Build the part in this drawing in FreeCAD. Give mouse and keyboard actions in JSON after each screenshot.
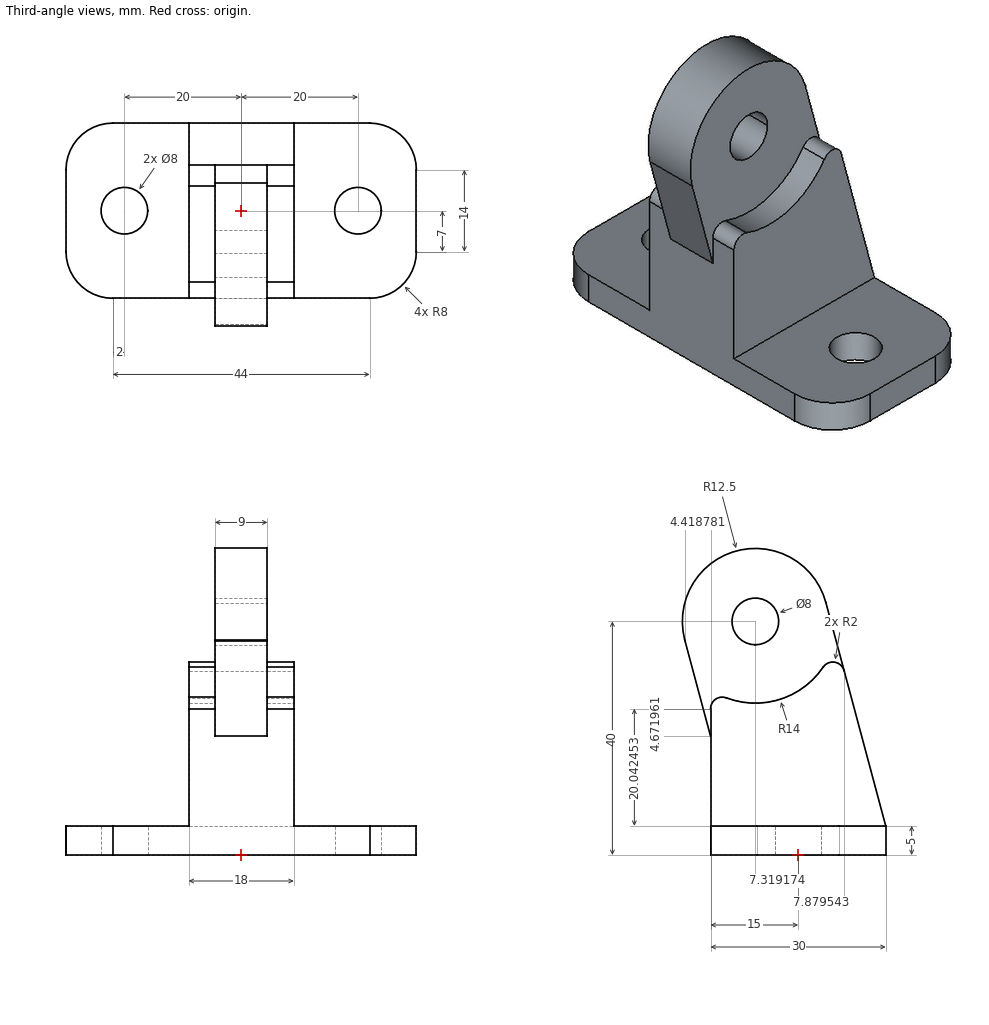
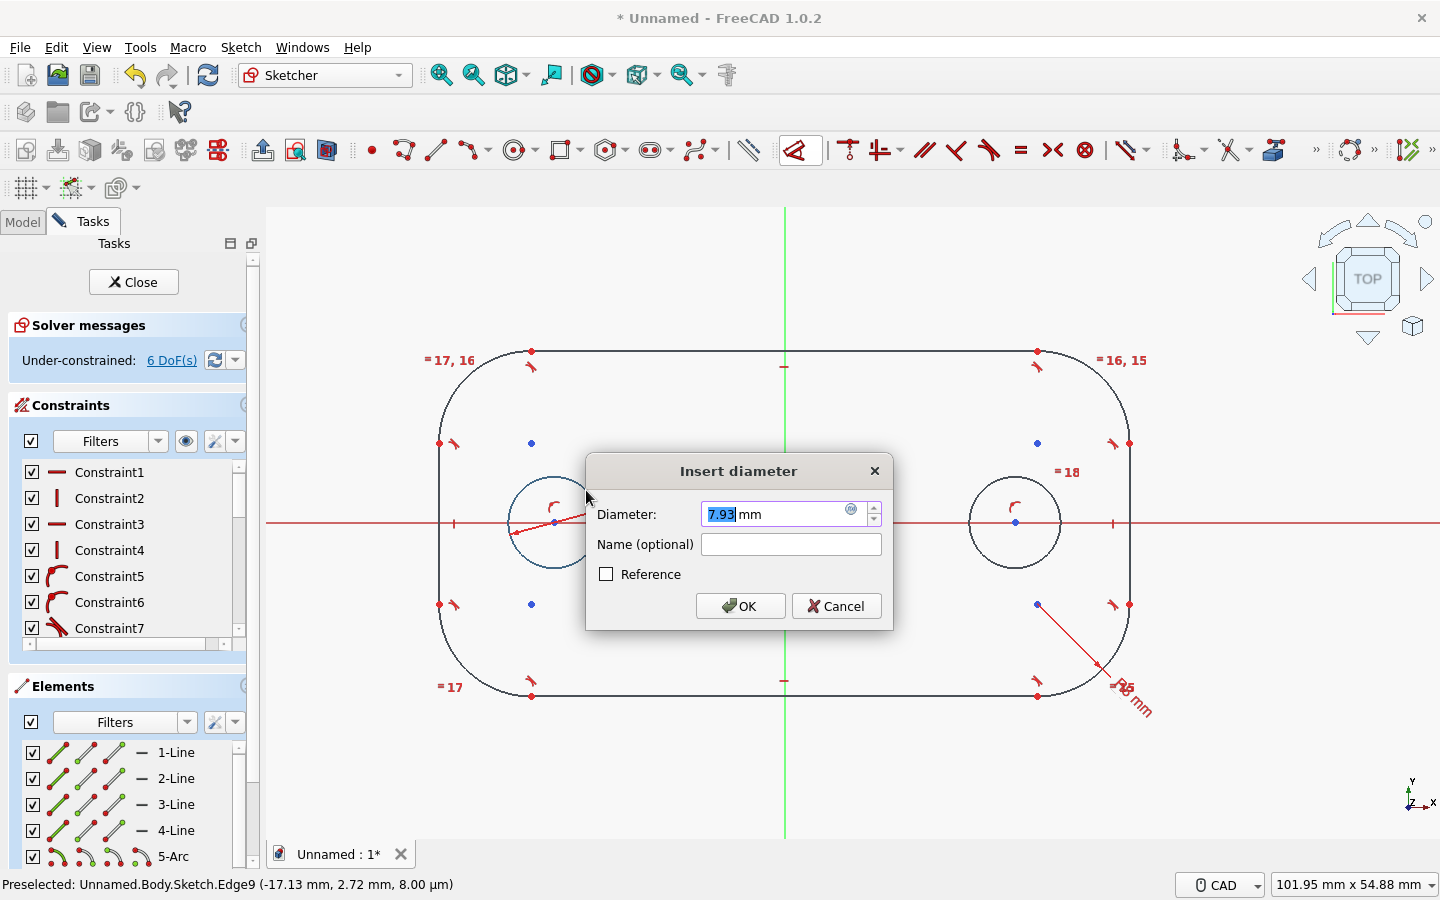
{"action": "type", "text": "8"}
{"action": "key", "text": "Return"}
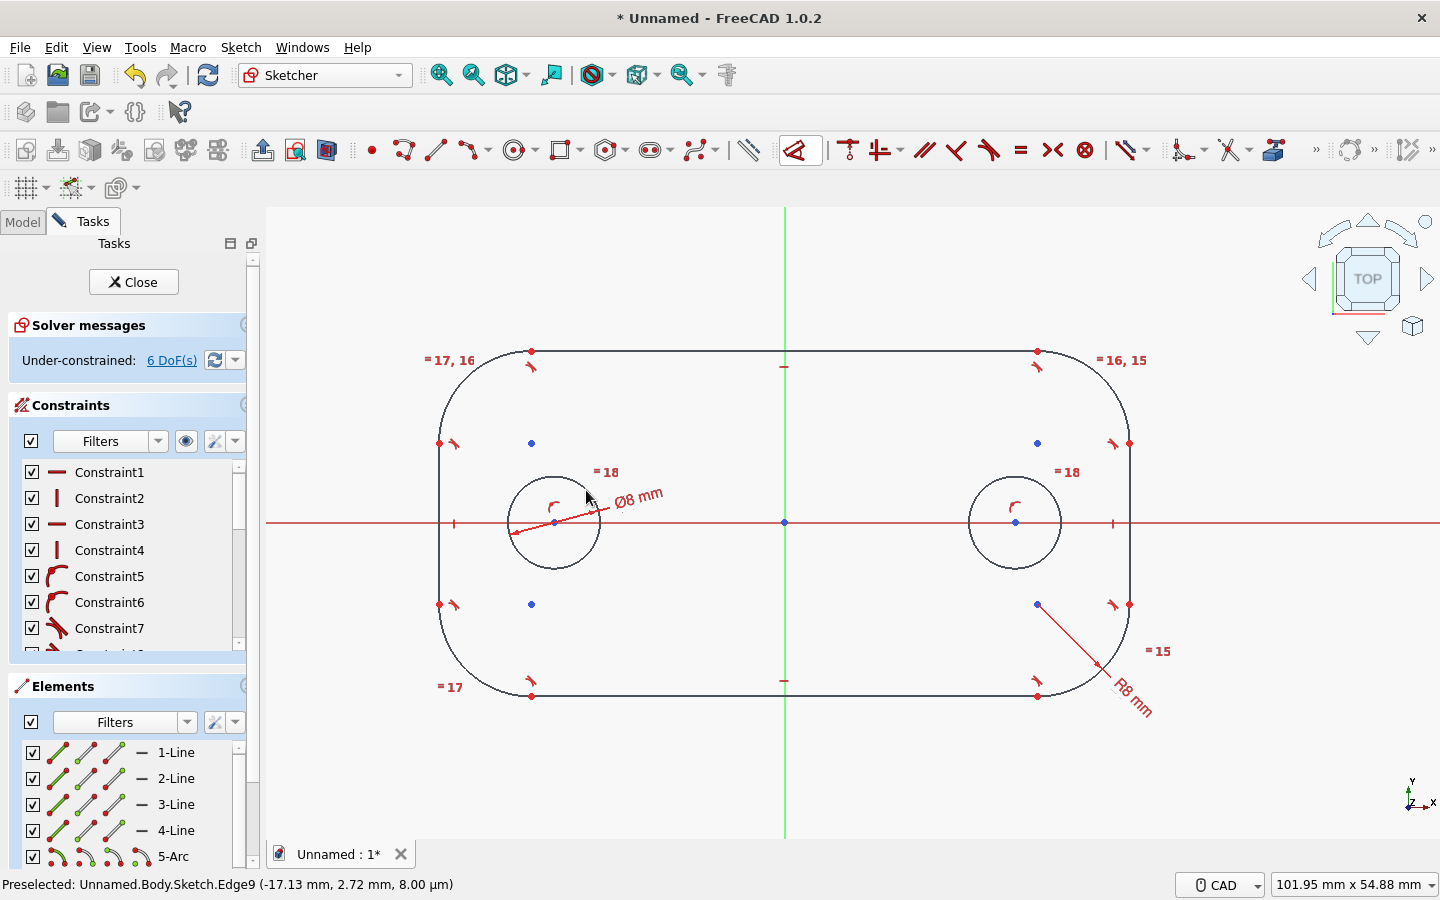
{"action": "left_click", "coordinate": [683, 696]}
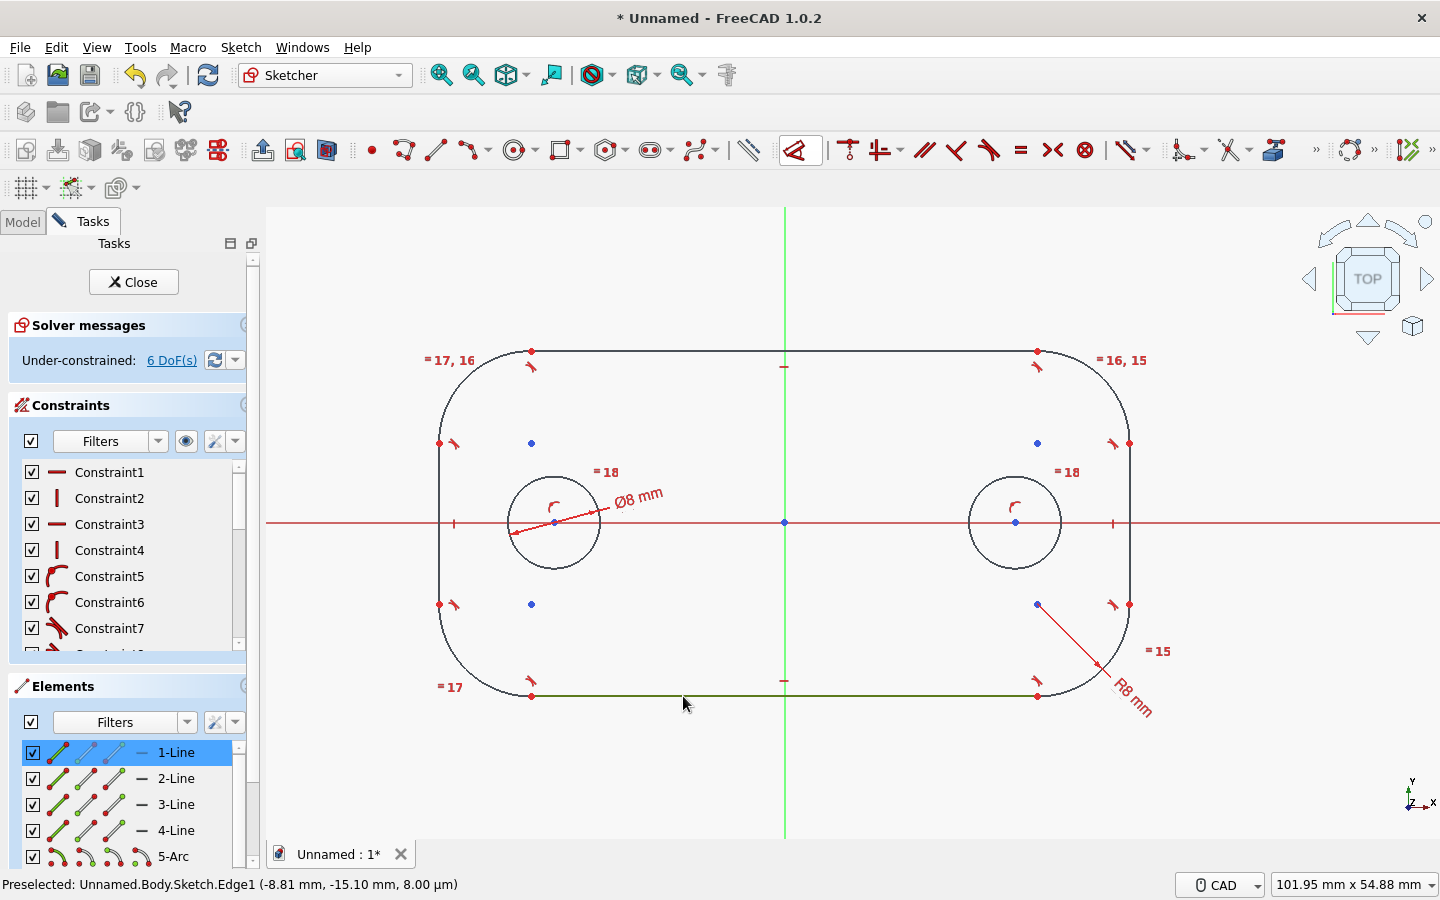
{"action": "key", "text": "l"}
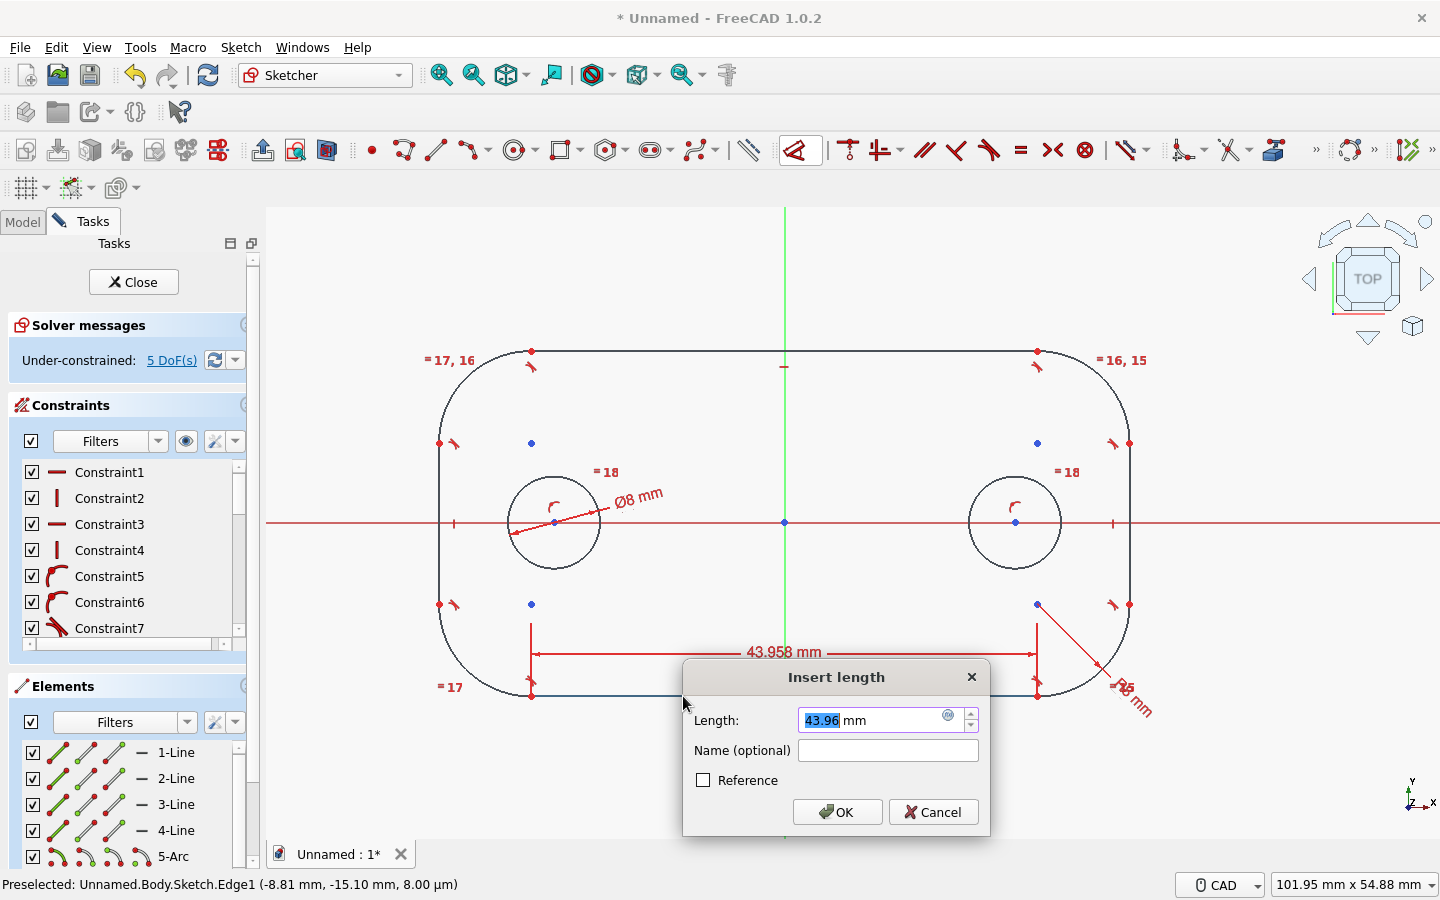
{"action": "type", "text": "44"}
{"action": "key", "text": "Return"}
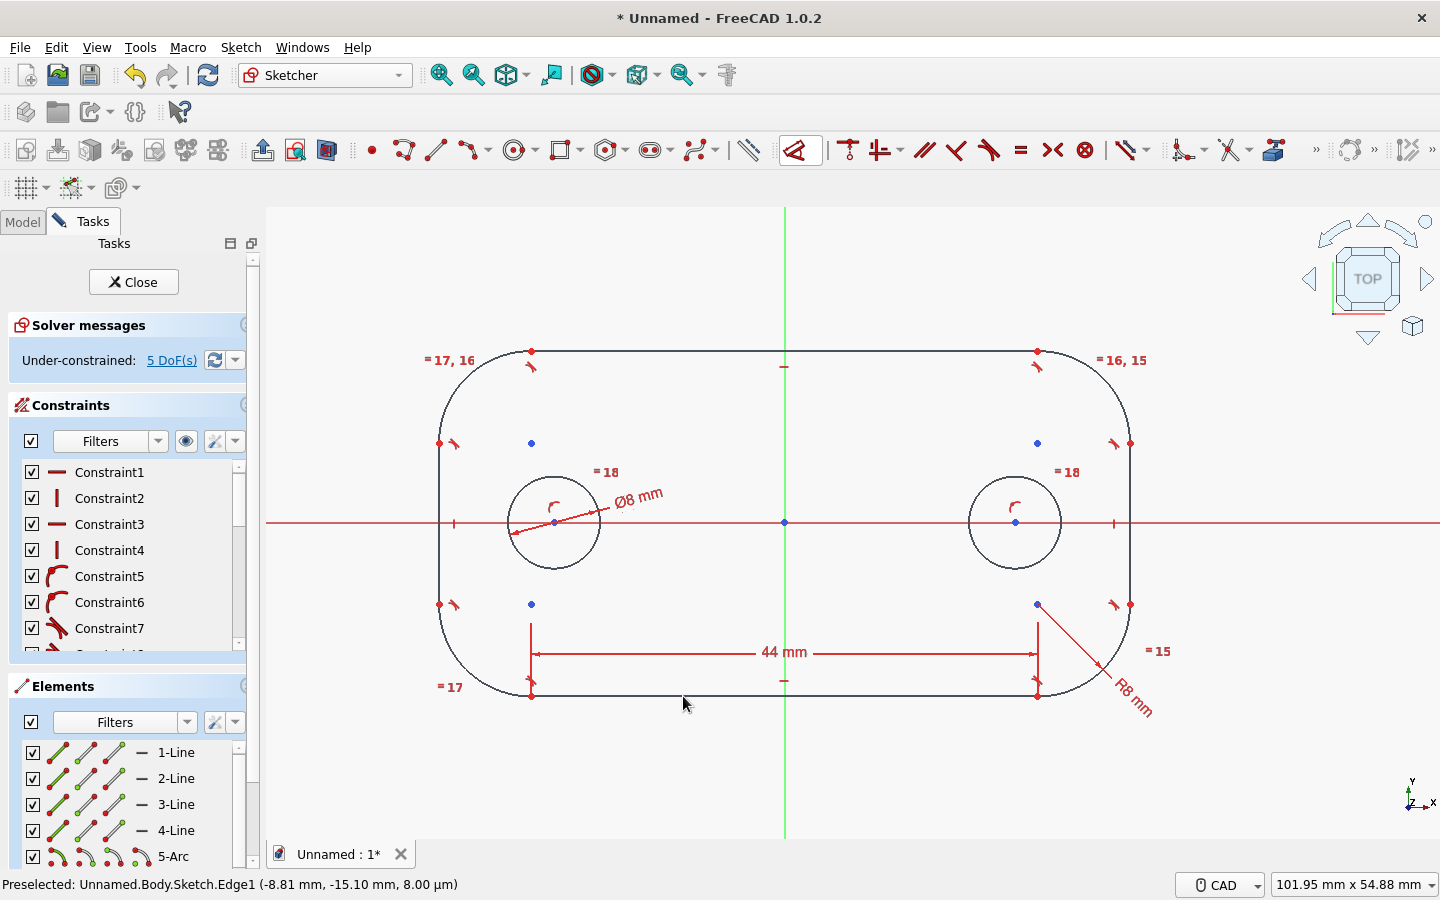
{"action": "left_click", "coordinate": [1130, 556]}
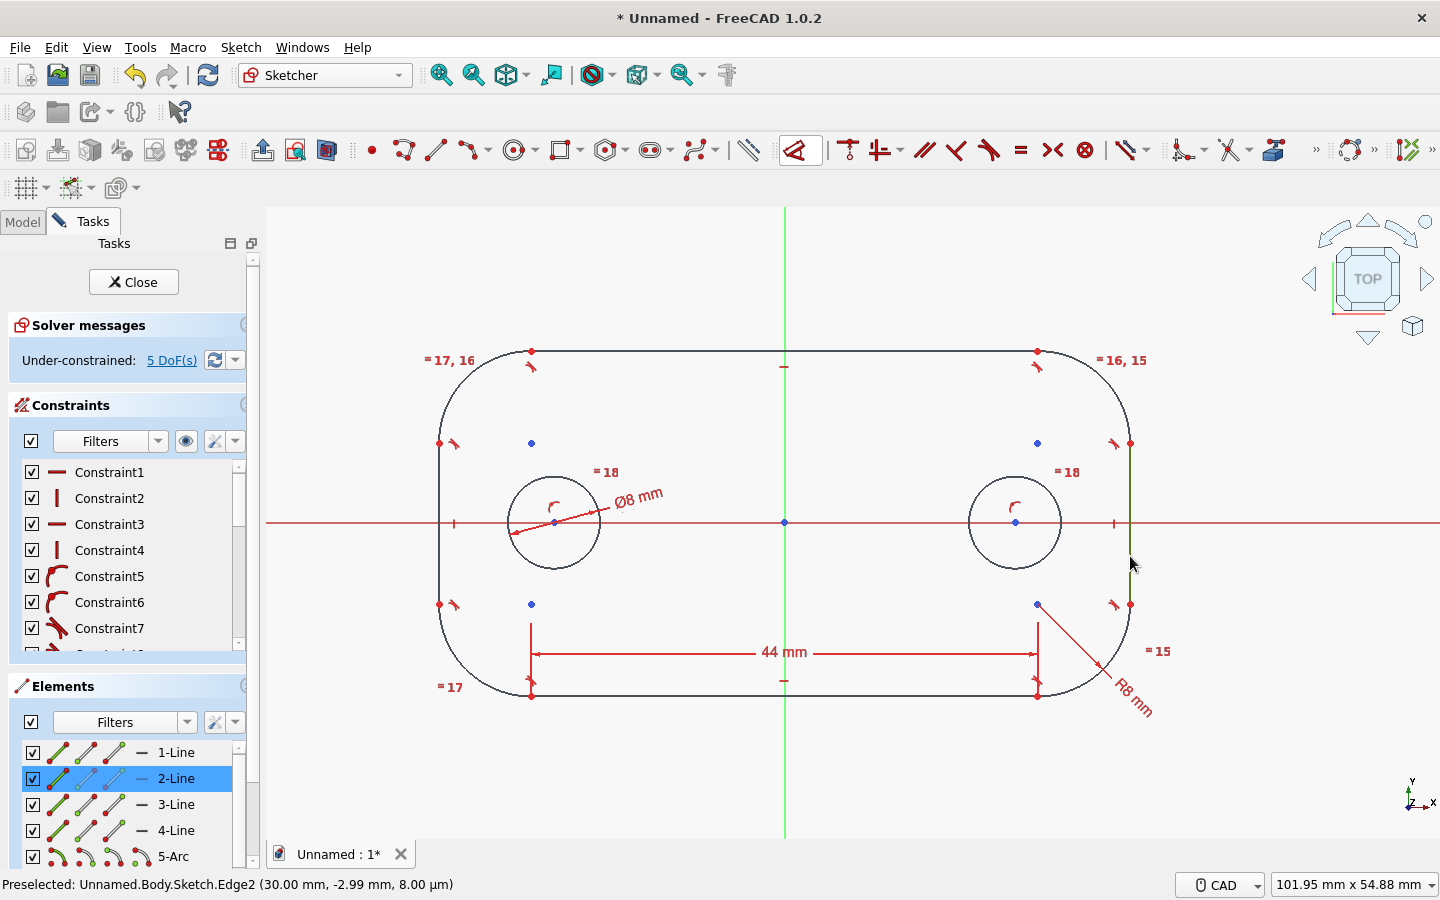
{"action": "key", "text": "i"}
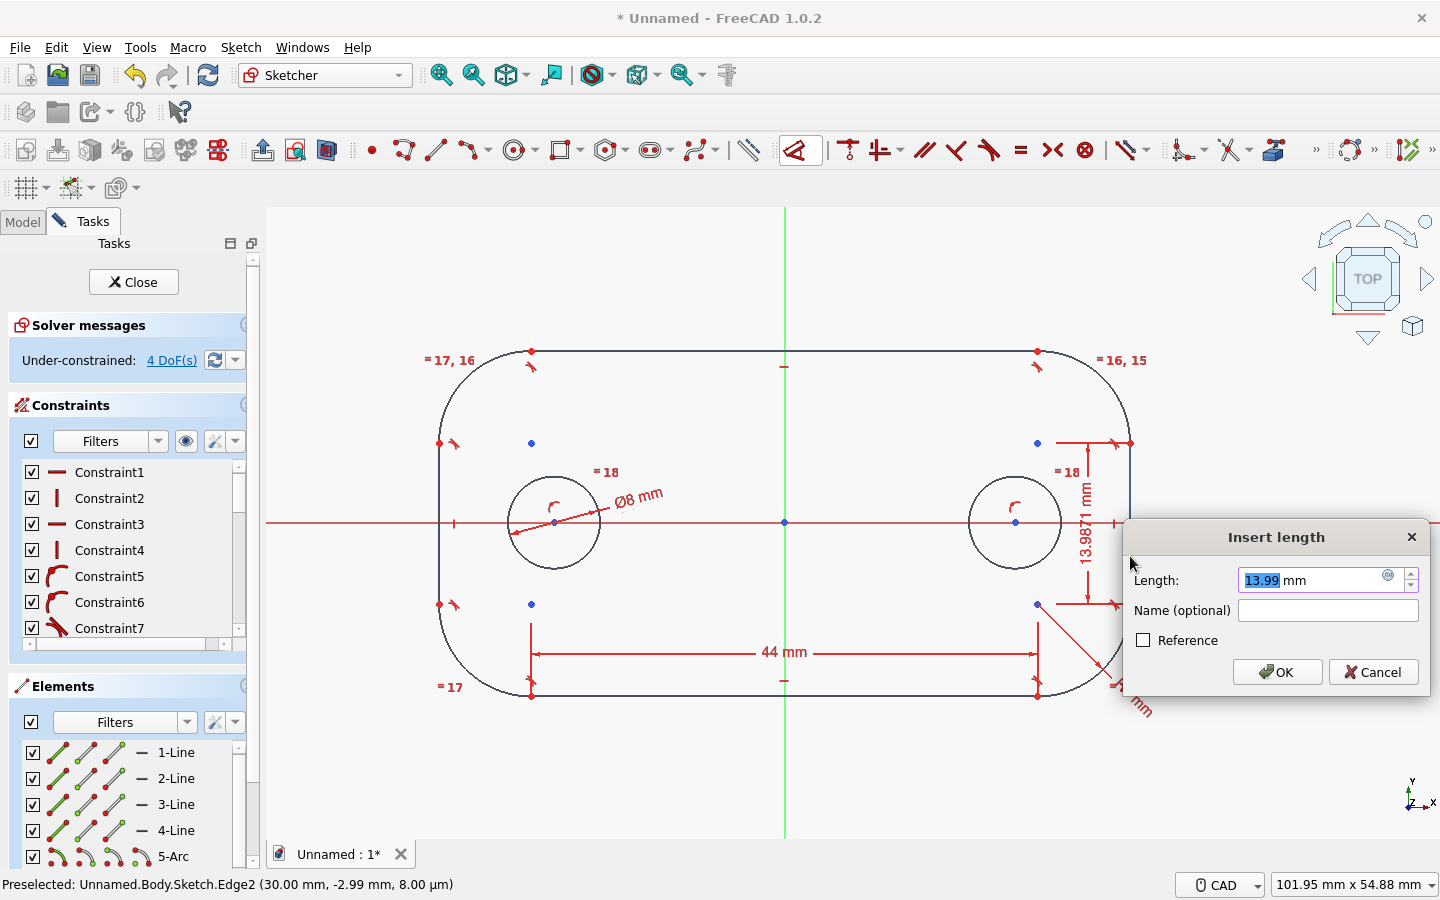
{"action": "type", "text": "14"}
{"action": "key", "text": "Return"}